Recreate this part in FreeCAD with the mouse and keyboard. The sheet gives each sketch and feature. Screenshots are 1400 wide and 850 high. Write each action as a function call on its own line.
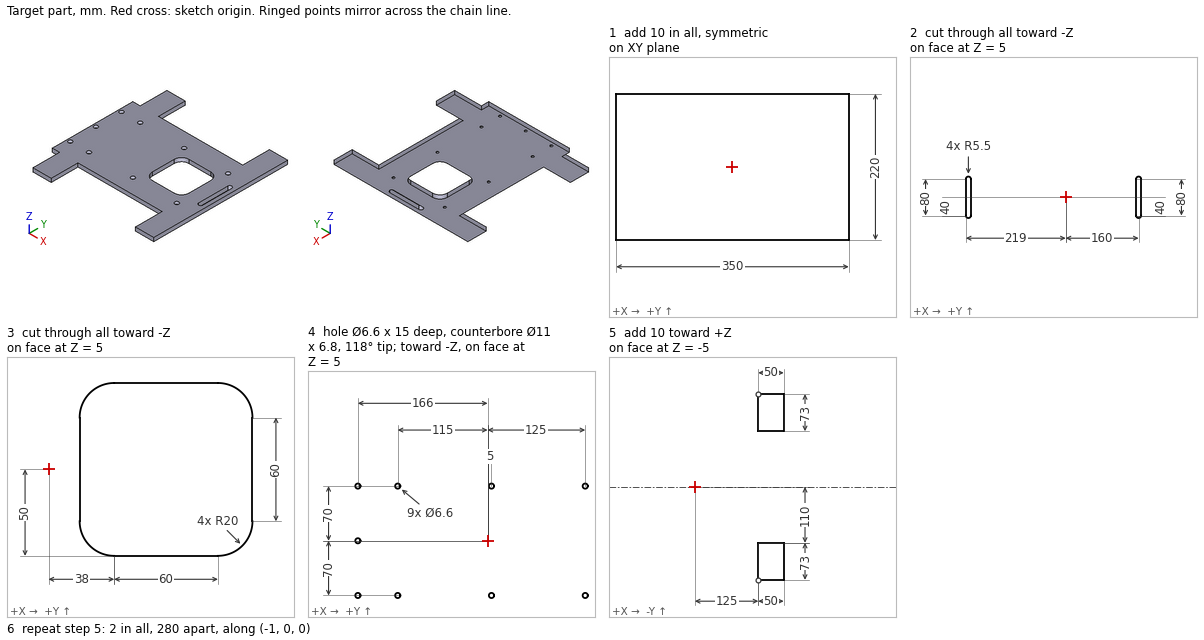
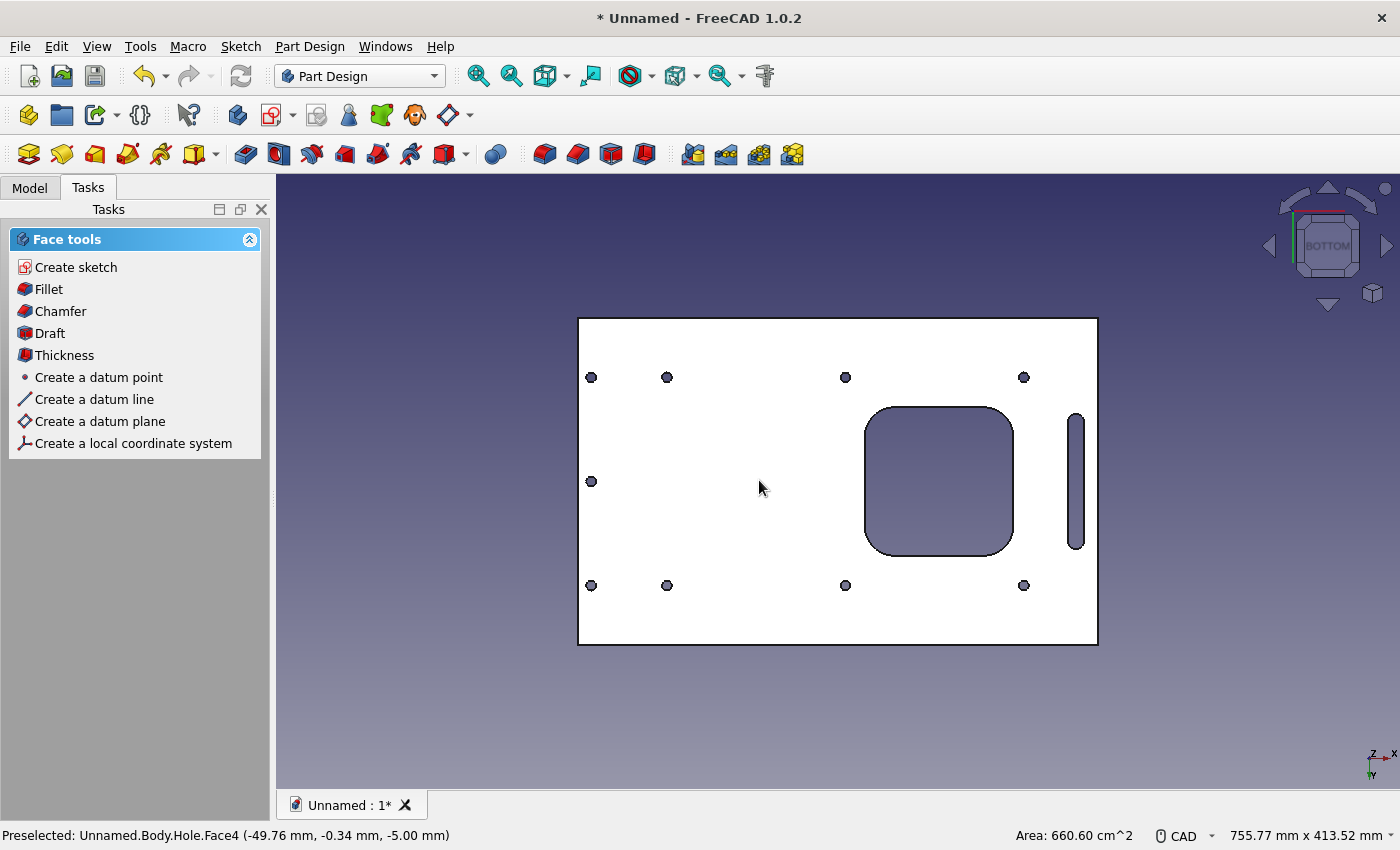
click(270, 116)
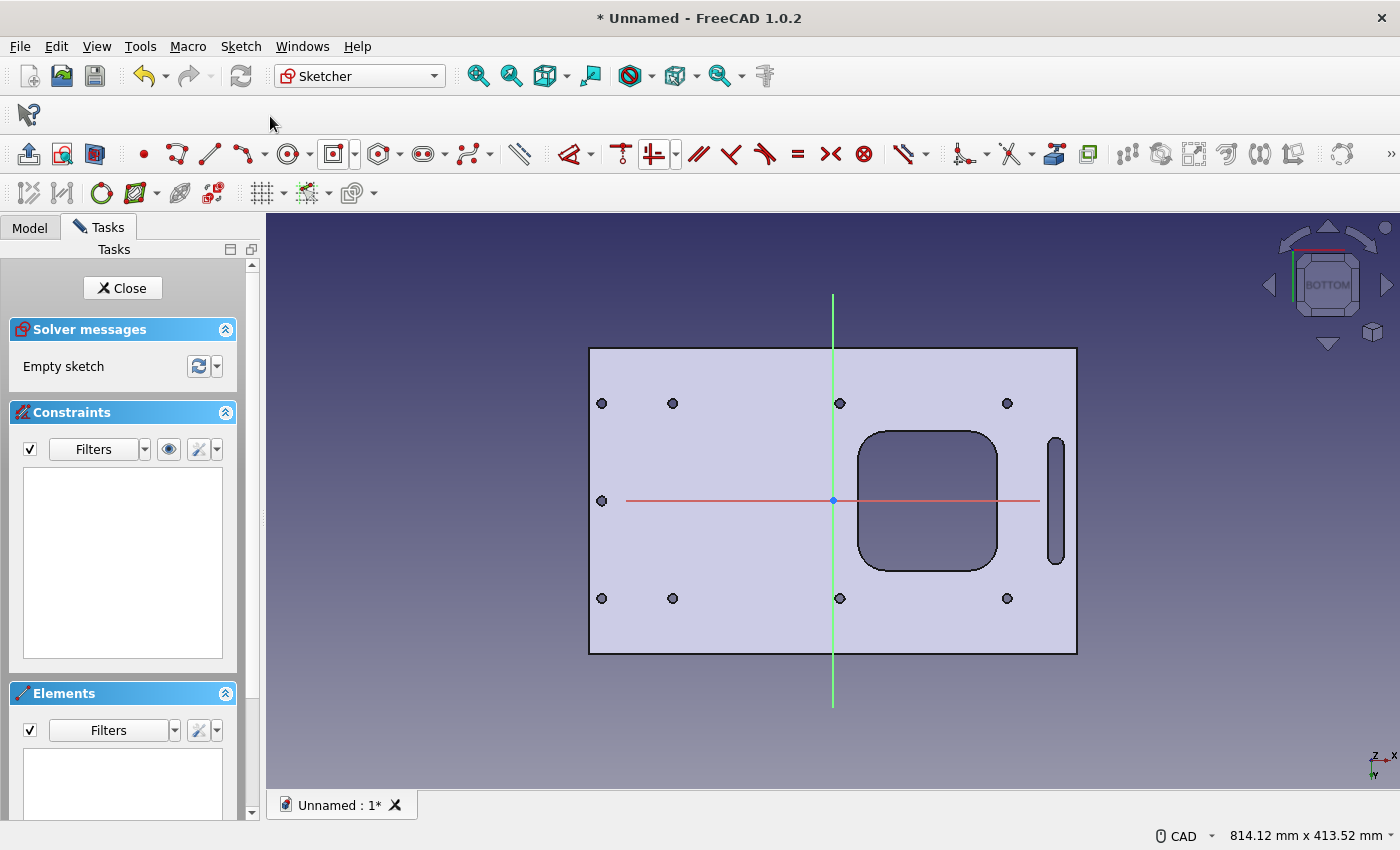
scroll(377, 501, down, 2)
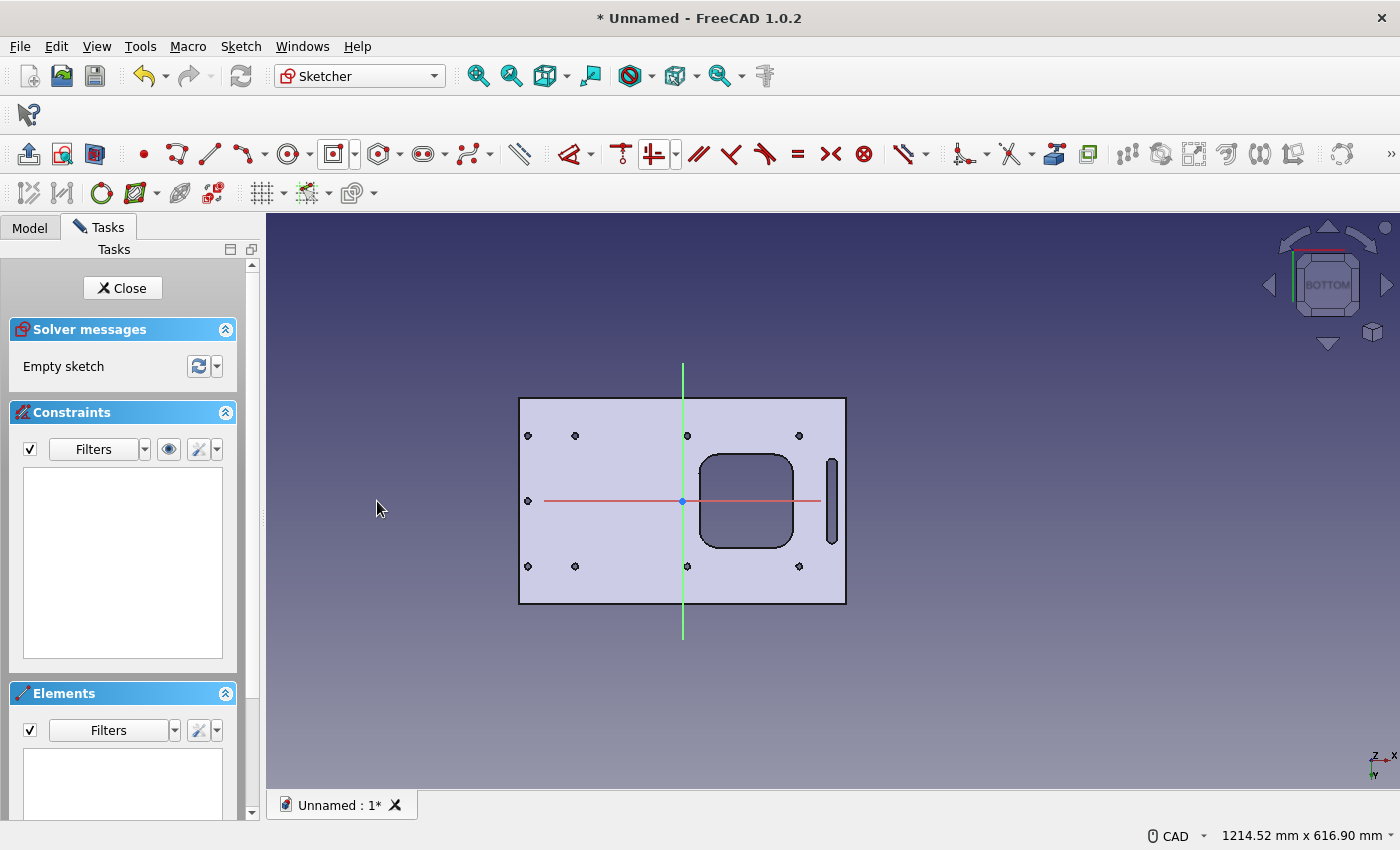
click(354, 154)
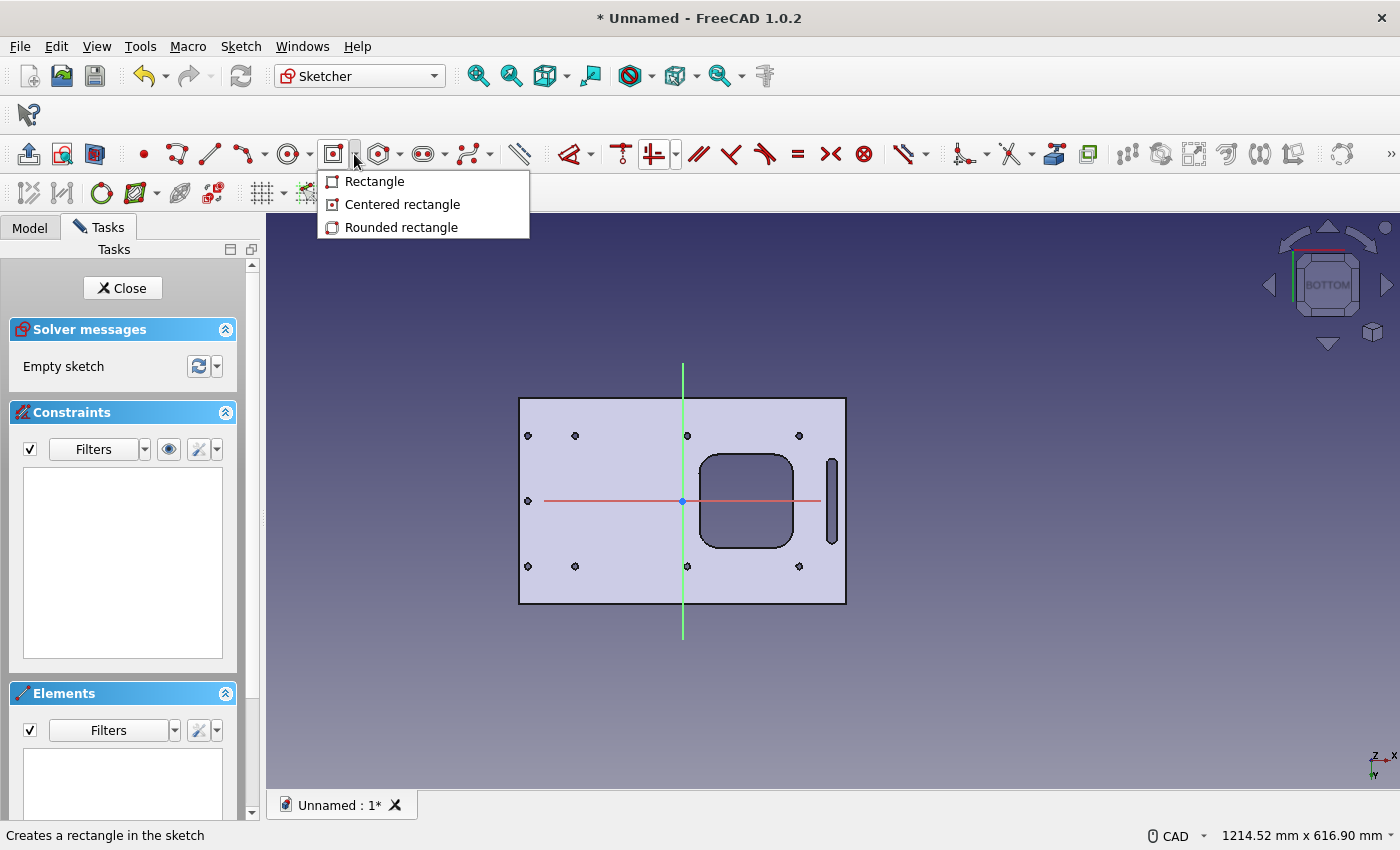
click(424, 182)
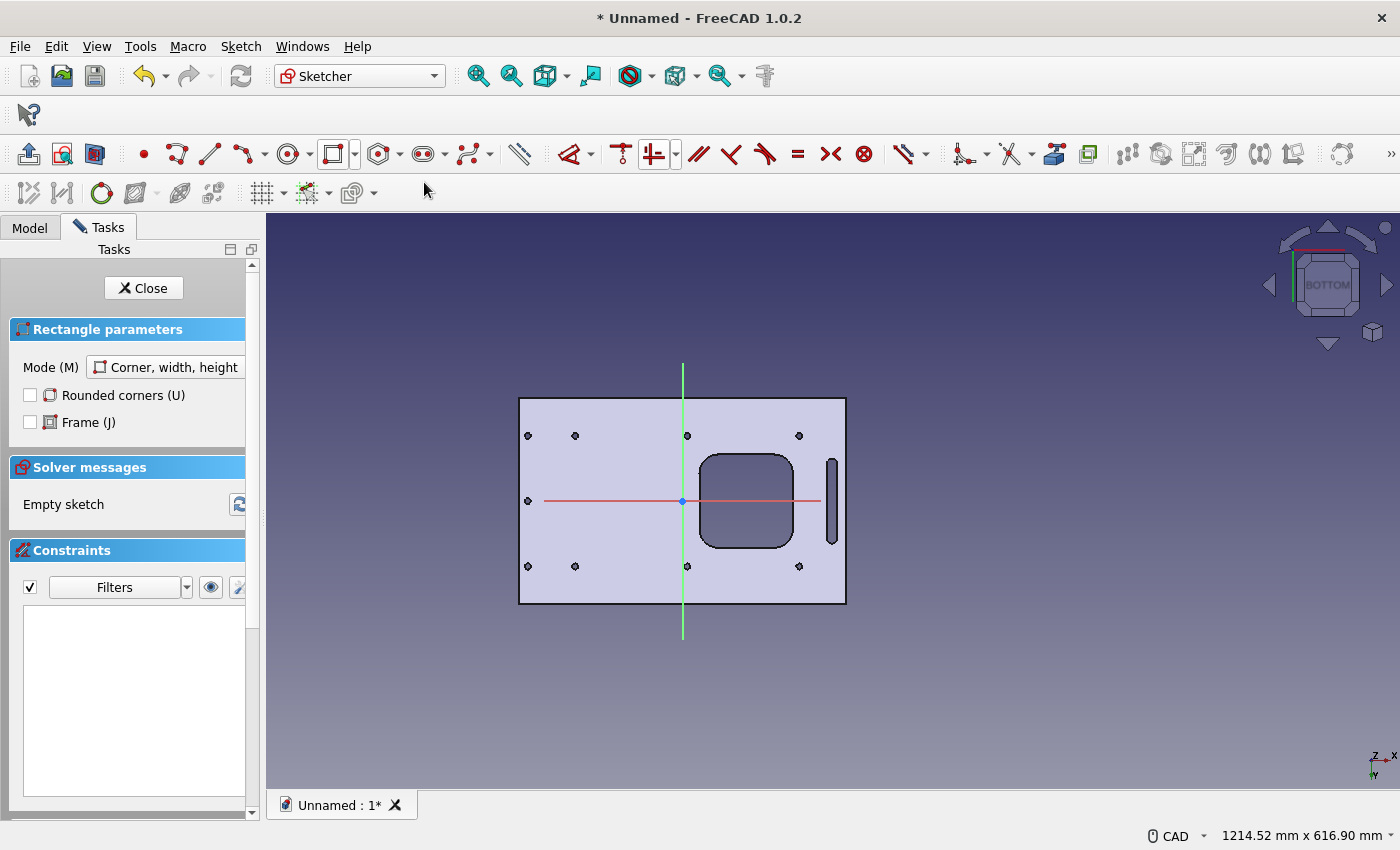
click(799, 604)
move(846, 672)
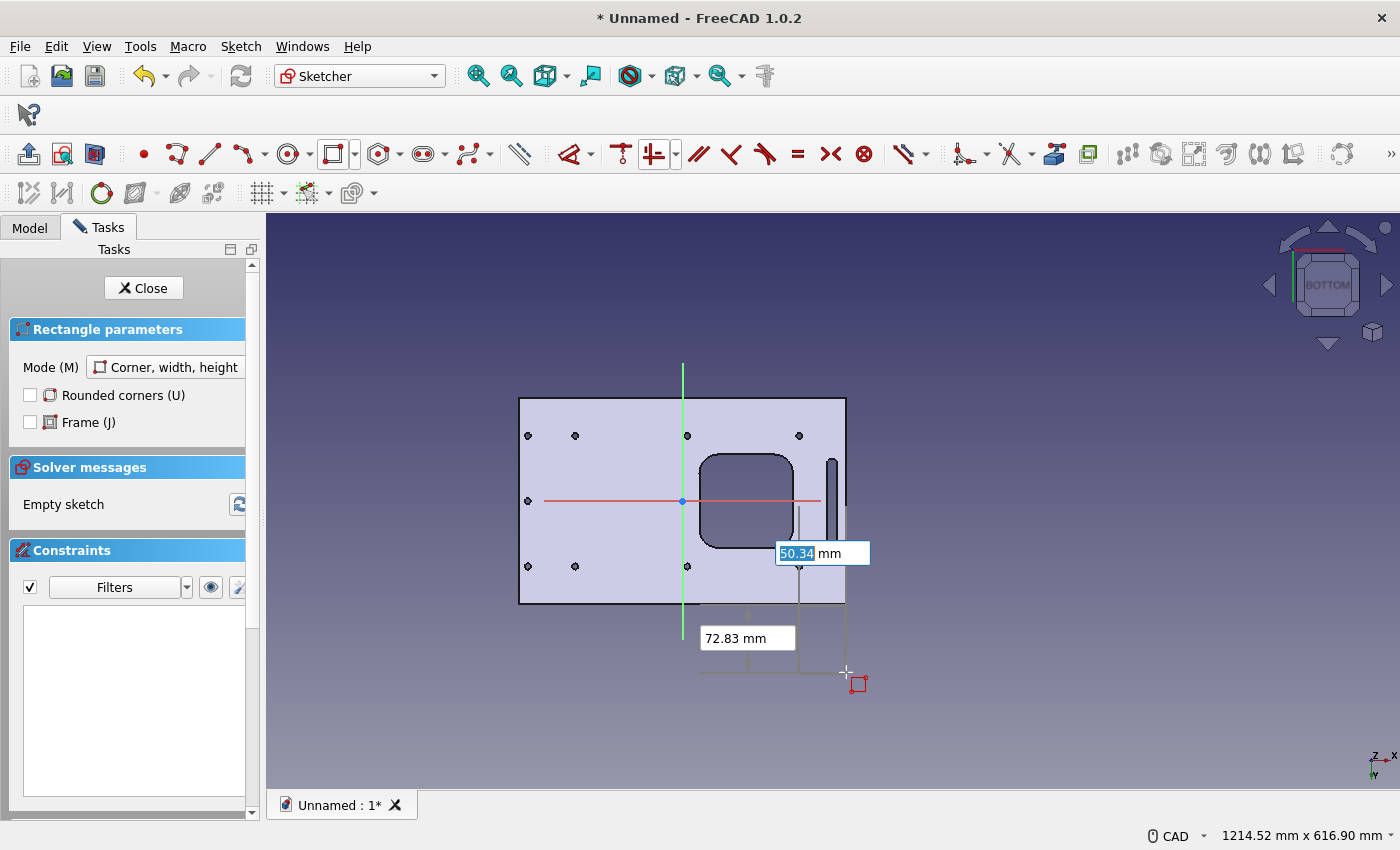
text(50)
key(Tab)
text(73)
key(Return)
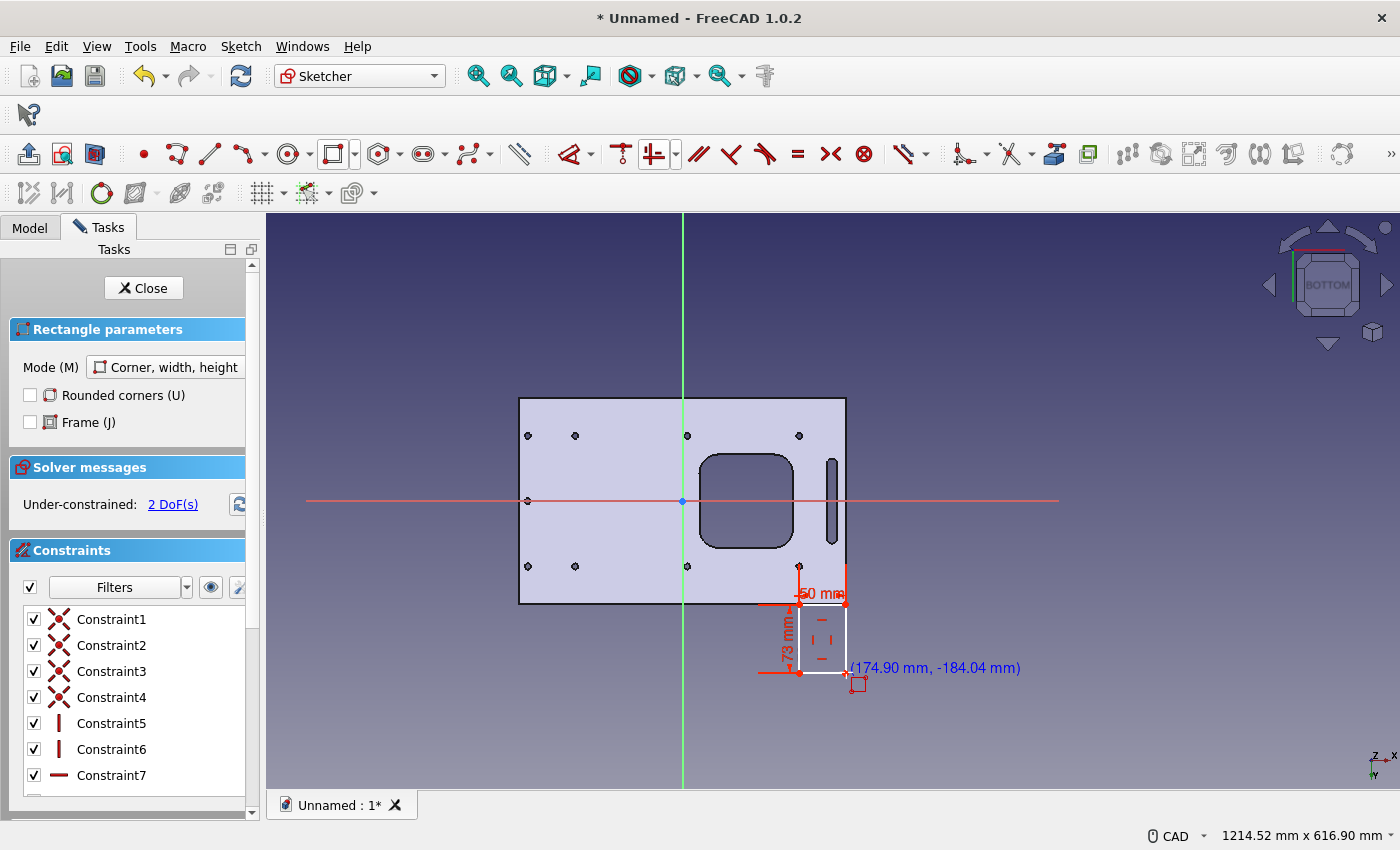
click(799, 330)
move(846, 398)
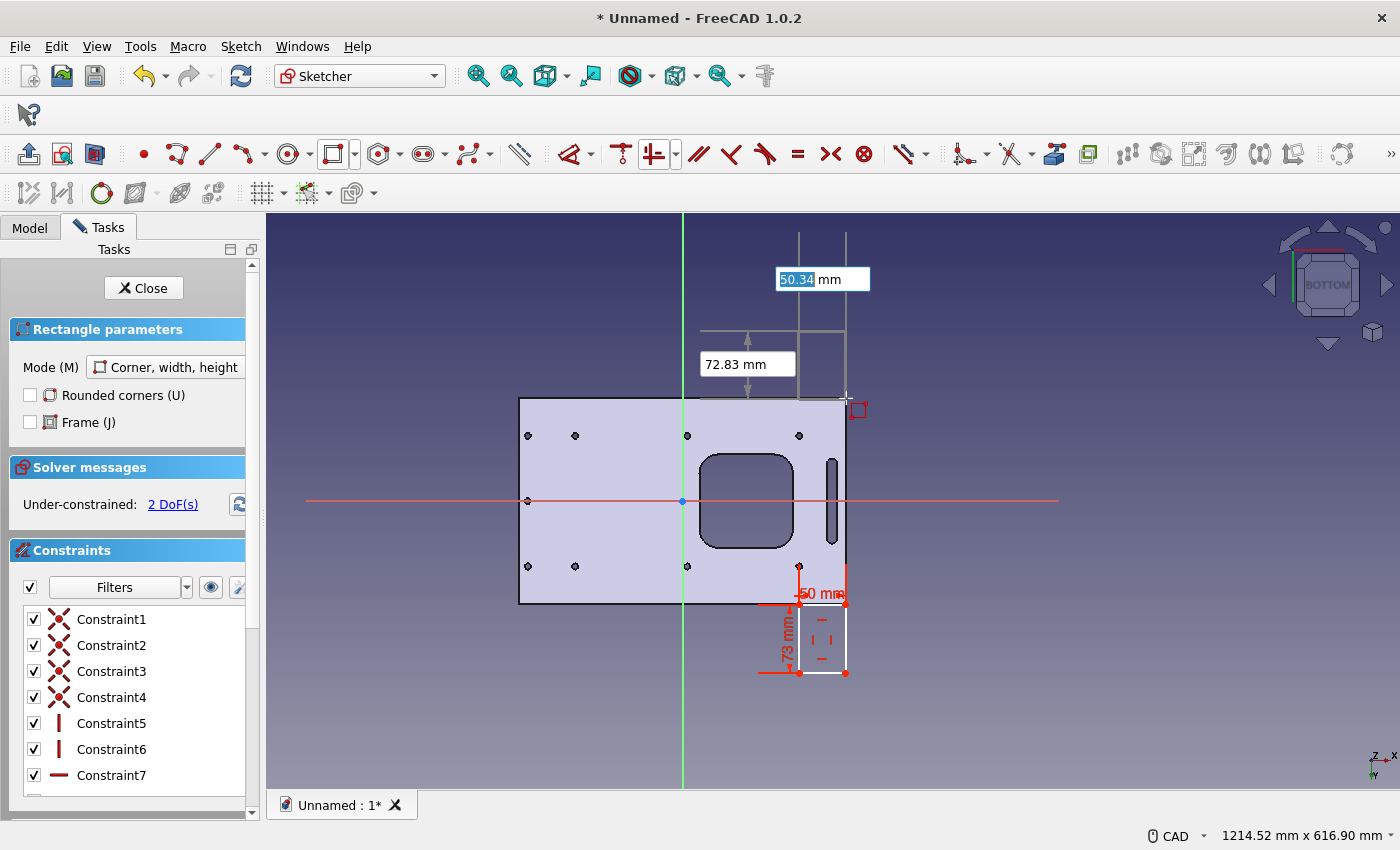
text(50)
key(Tab)
text(73)
key(Return)
key(Escape)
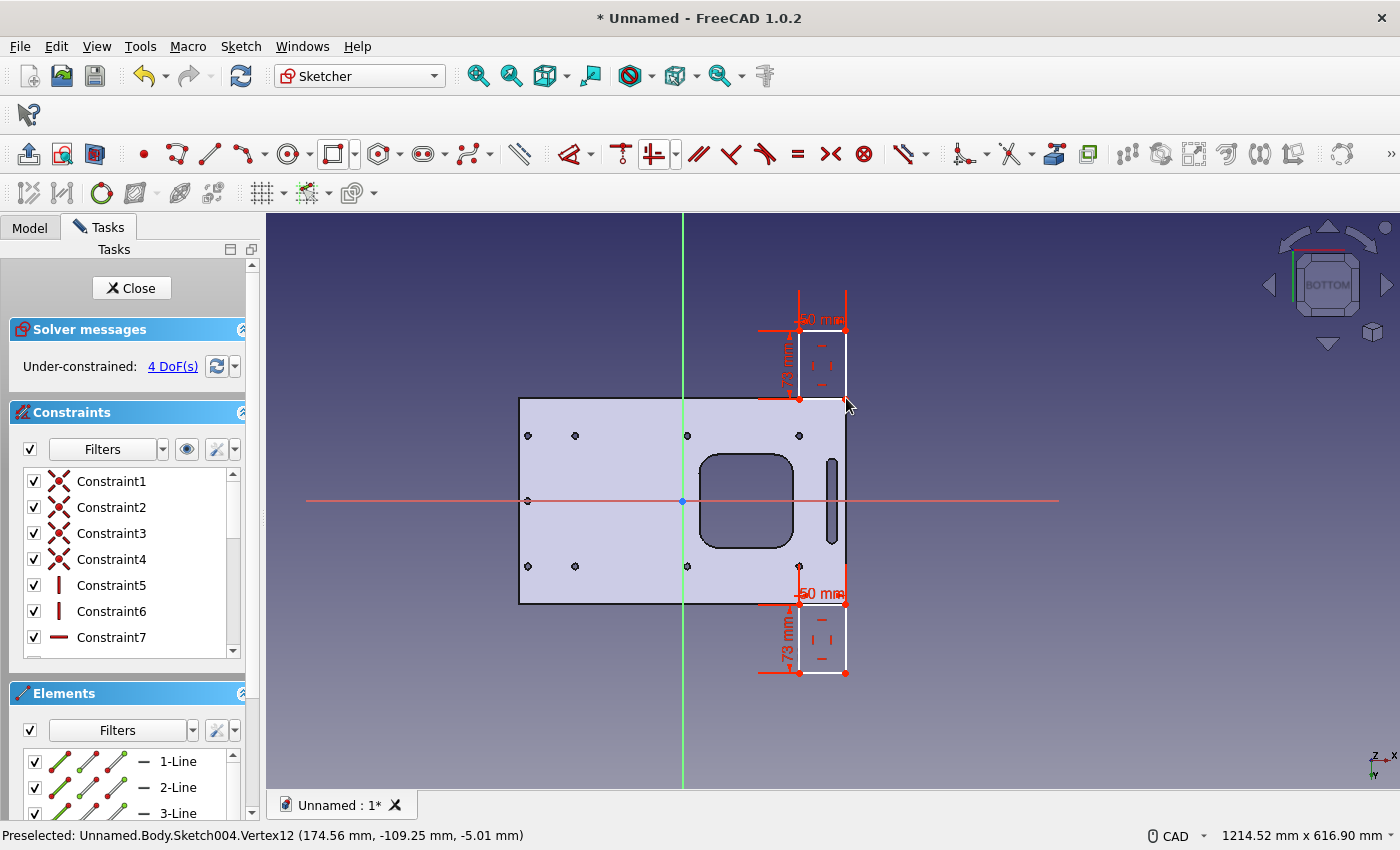
click(799, 673)